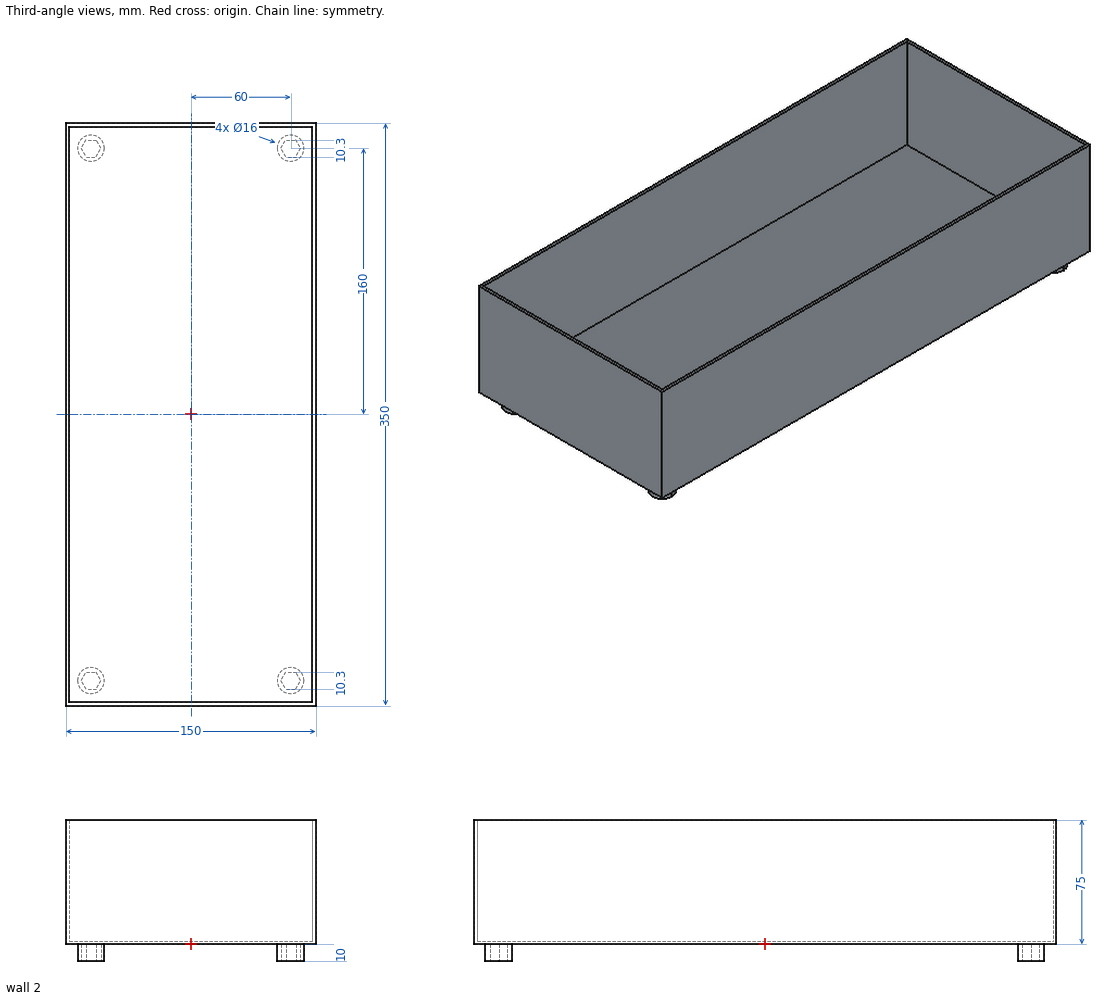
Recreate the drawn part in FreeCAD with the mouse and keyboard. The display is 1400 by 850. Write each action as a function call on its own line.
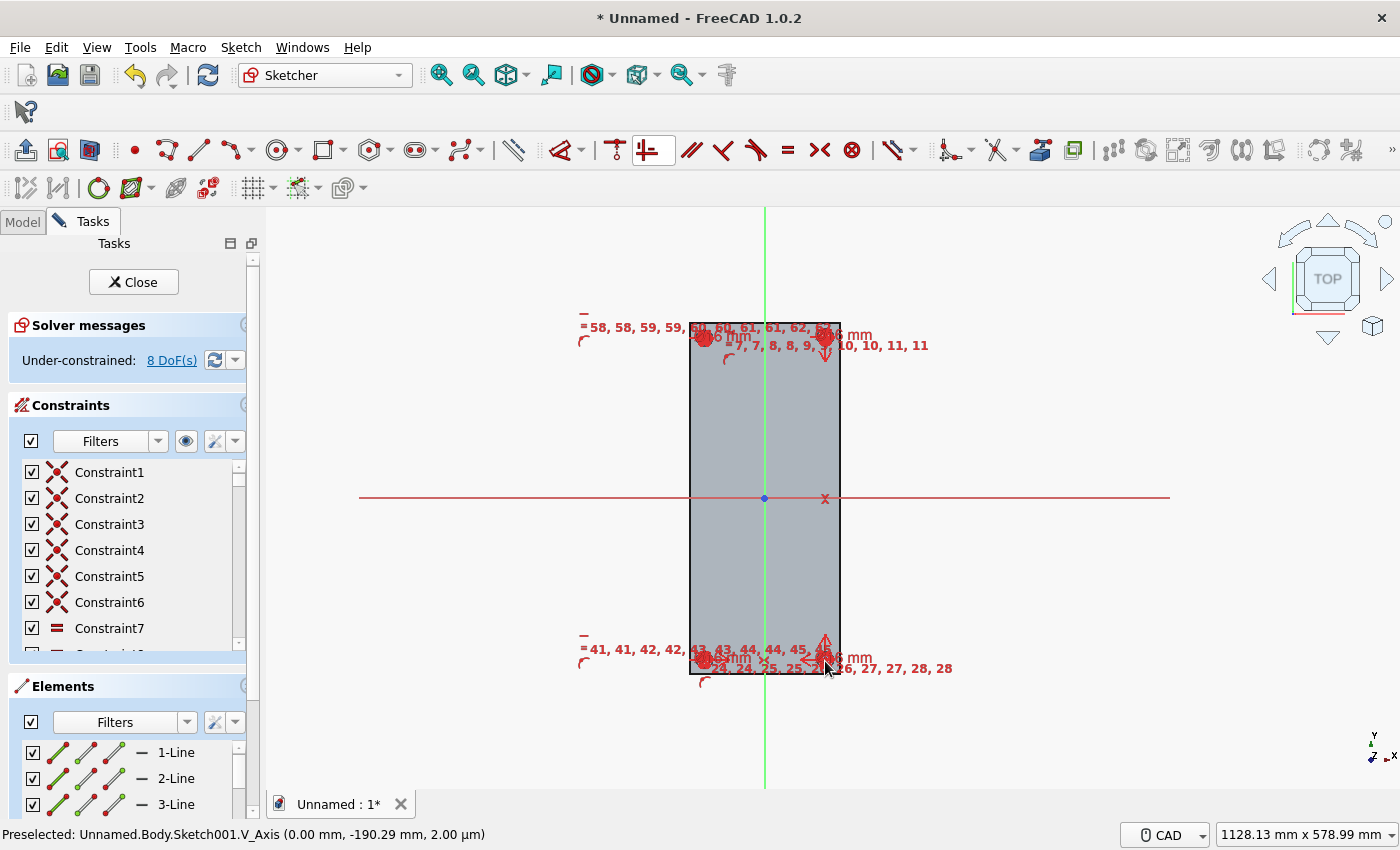
scroll(825, 337, up, 4)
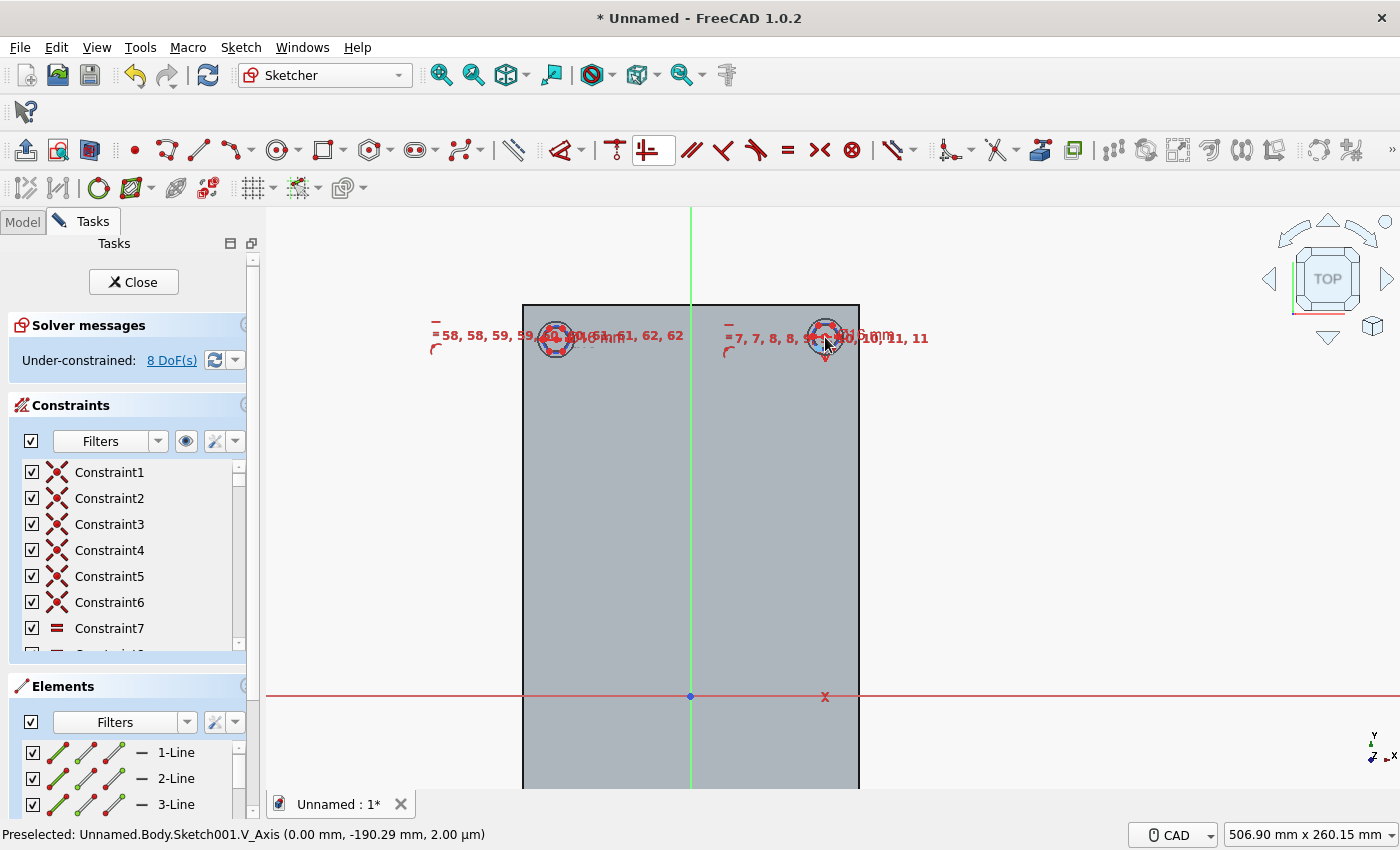
click(825, 337)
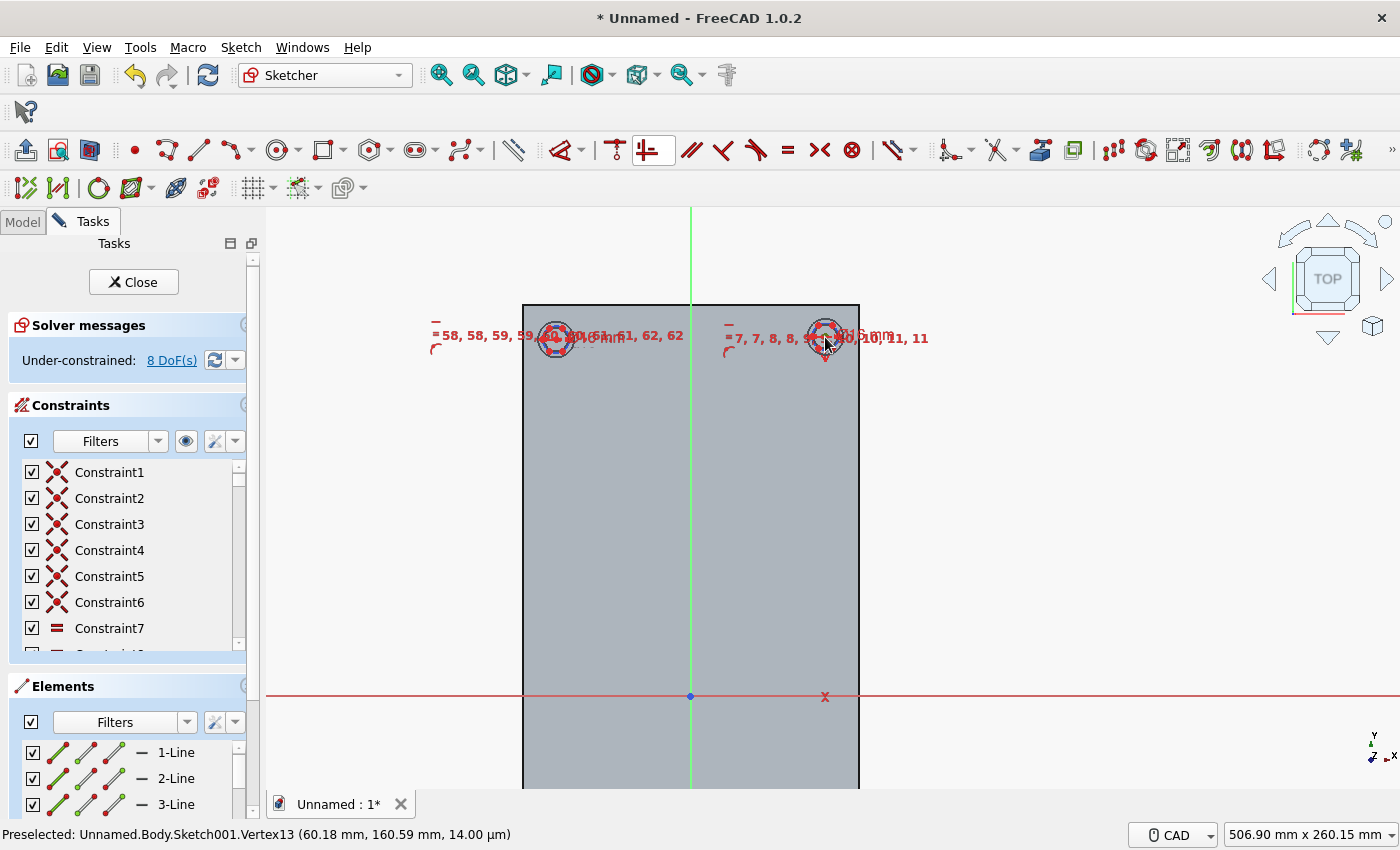
click(556, 340)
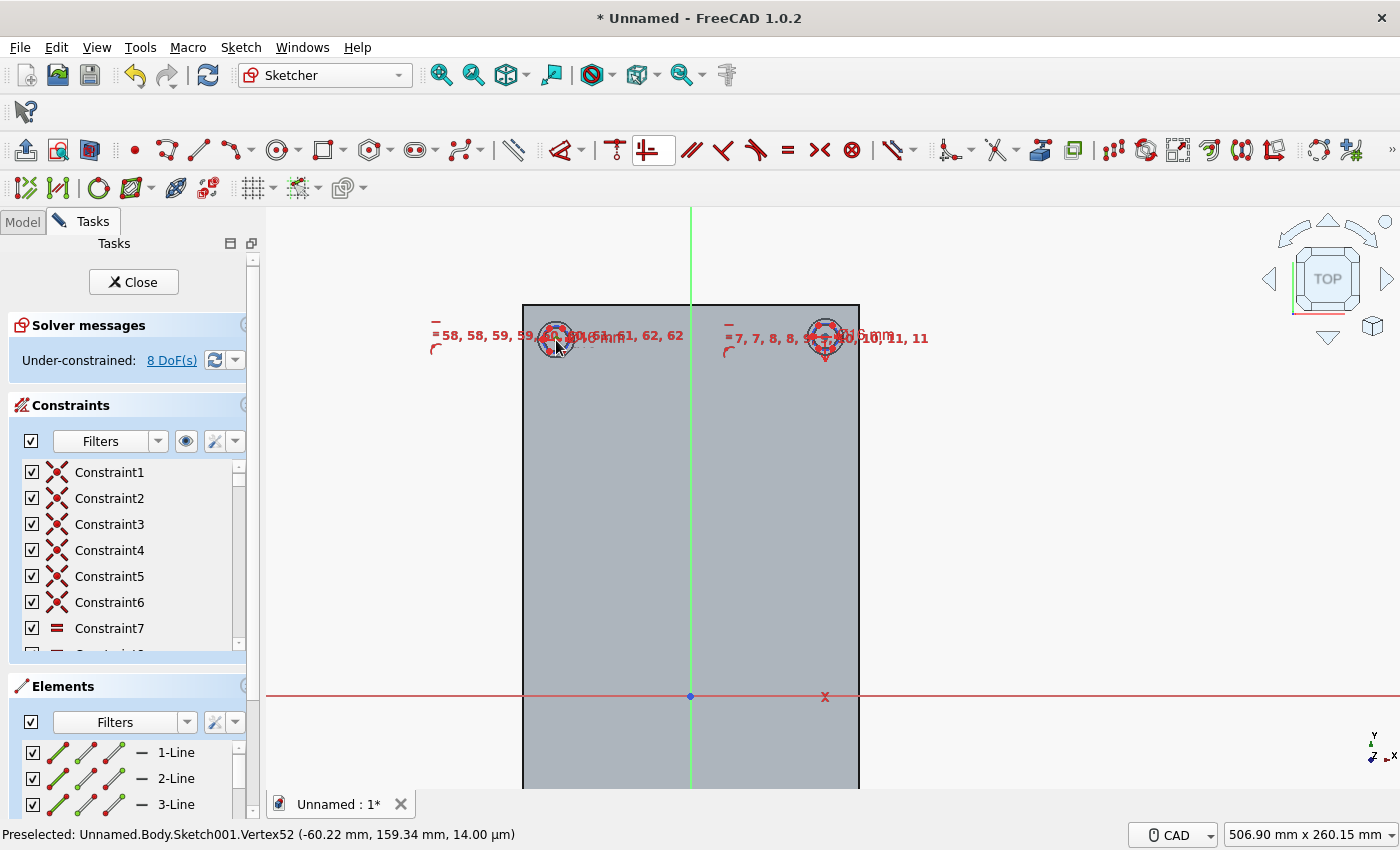
click(691, 648)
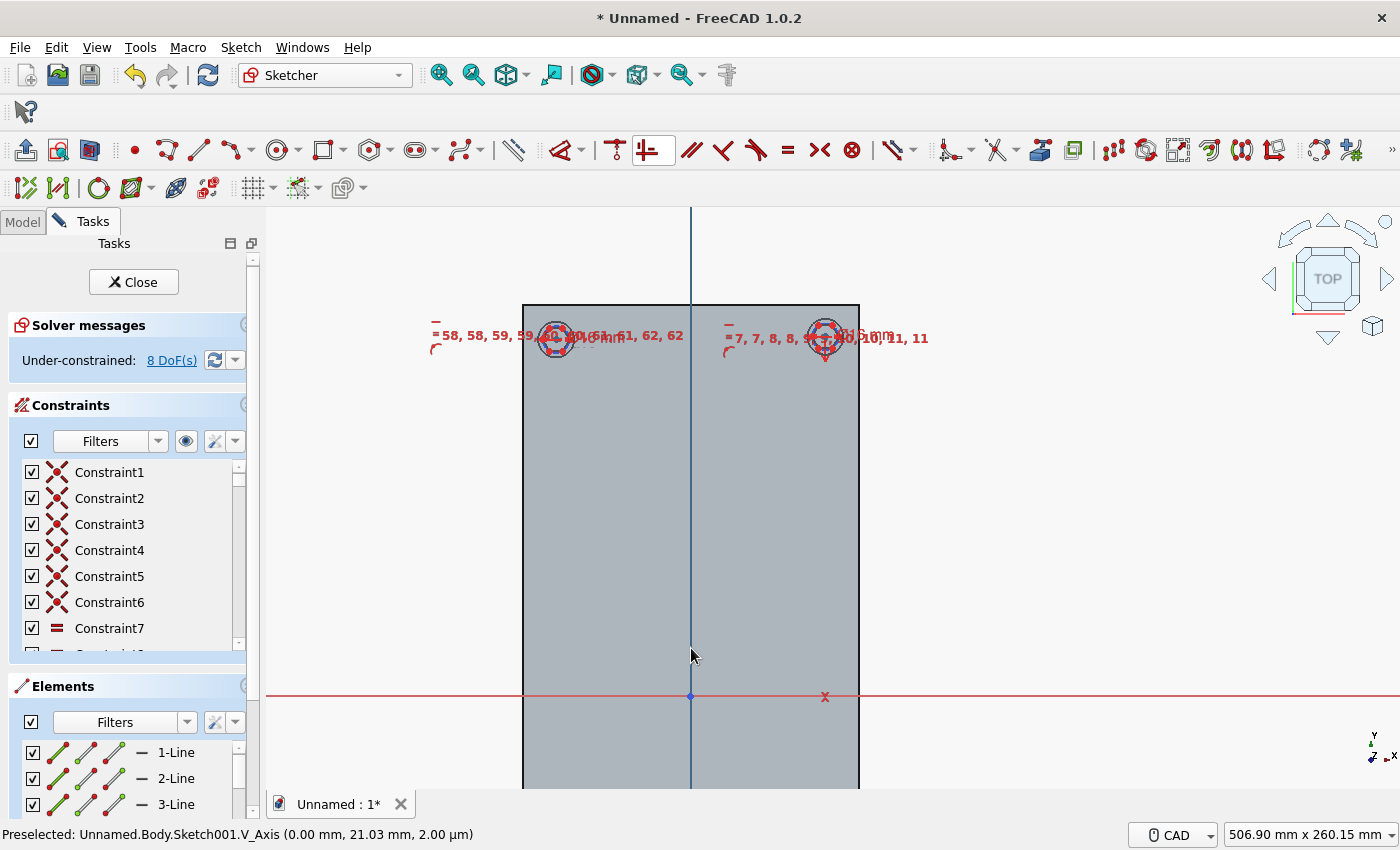
click(820, 150)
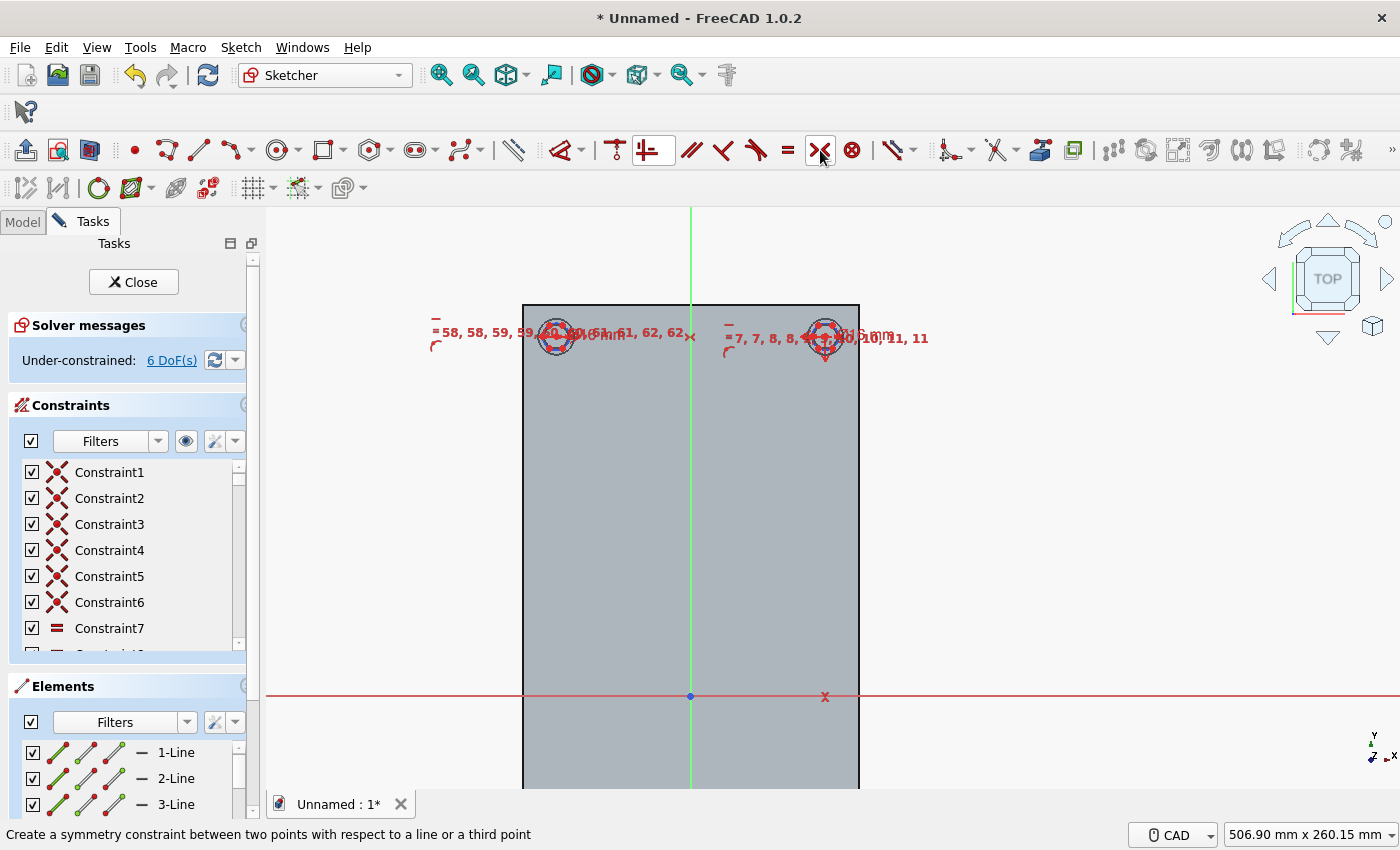
click(560, 150)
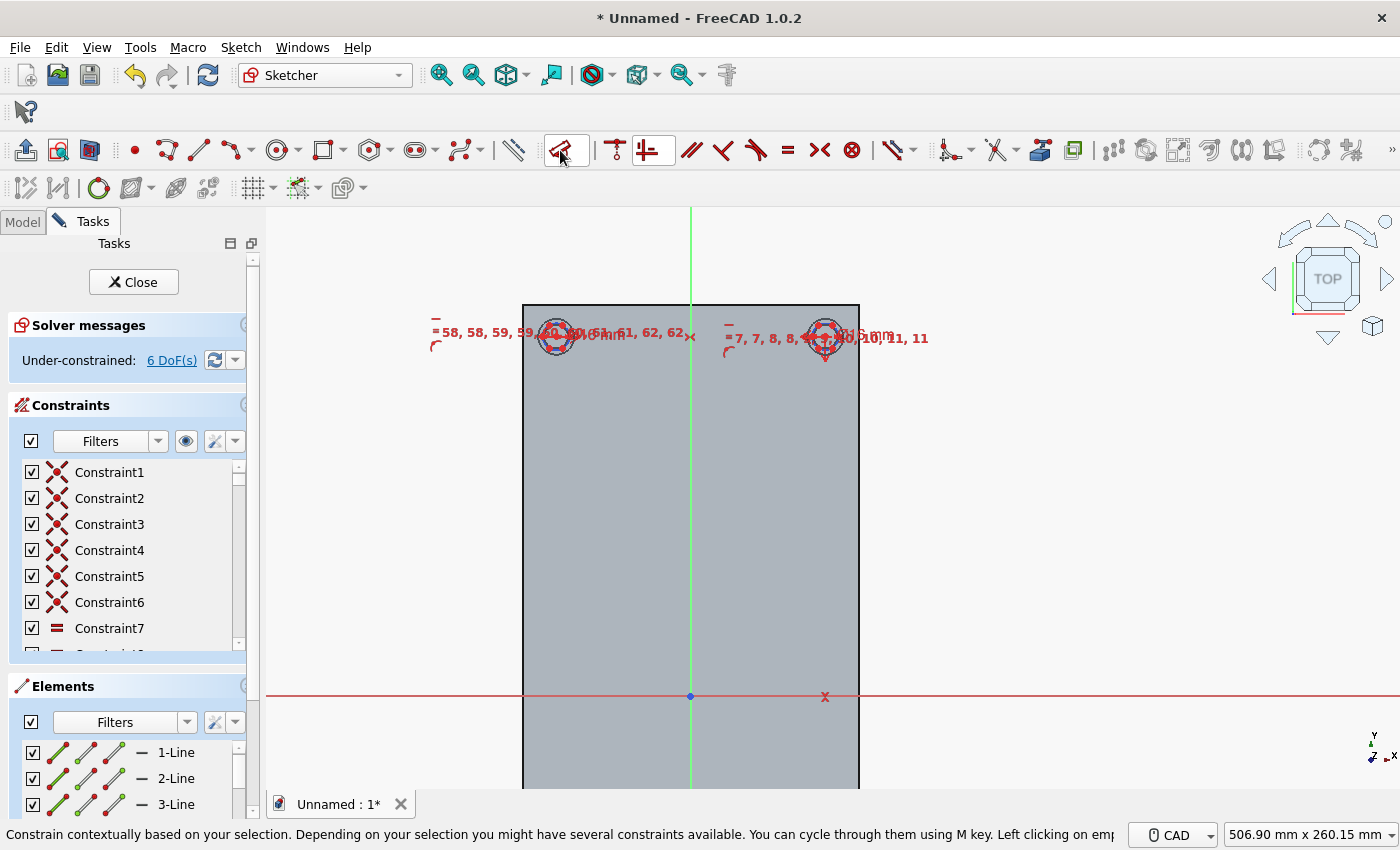
click(825, 337)
click(758, 303)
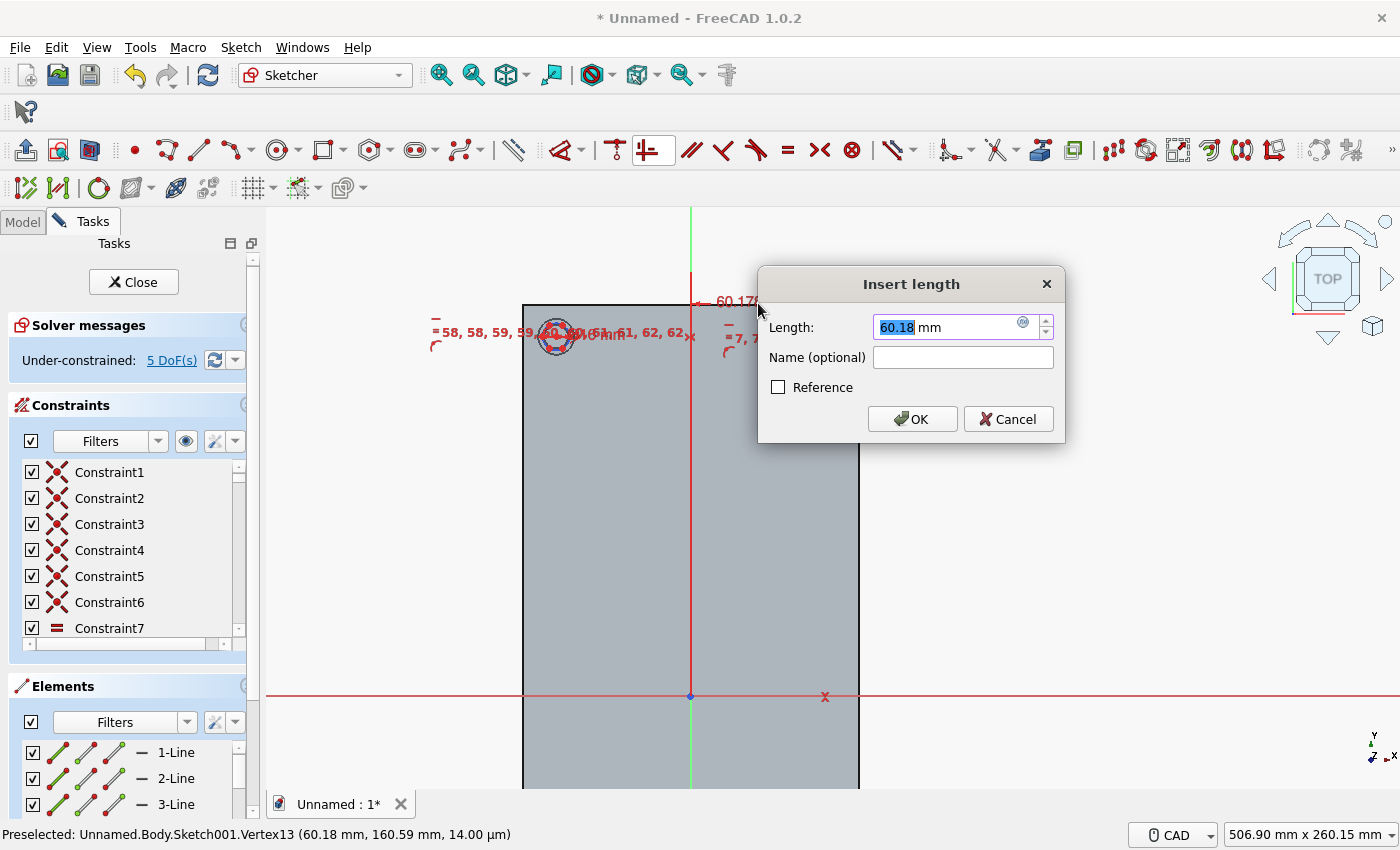
text(60)
key(Return)